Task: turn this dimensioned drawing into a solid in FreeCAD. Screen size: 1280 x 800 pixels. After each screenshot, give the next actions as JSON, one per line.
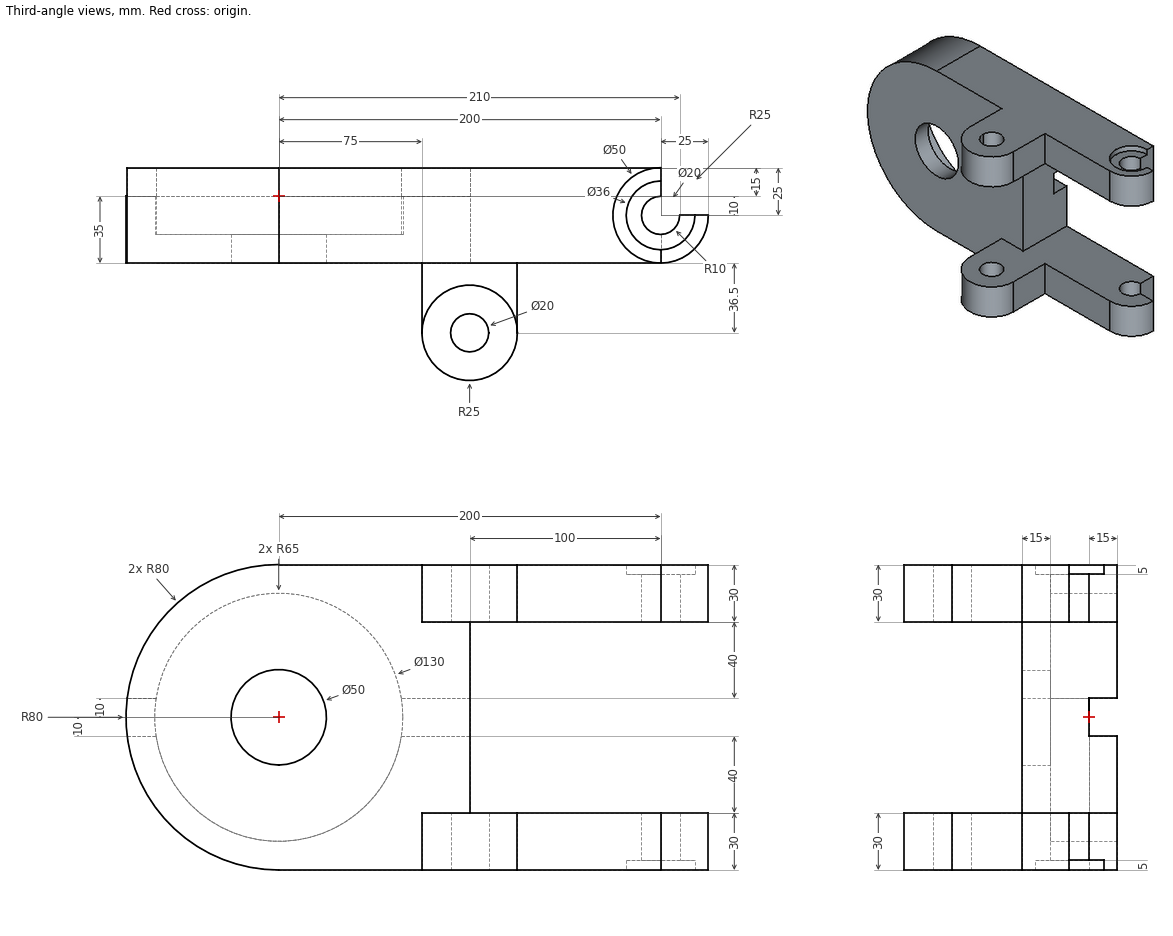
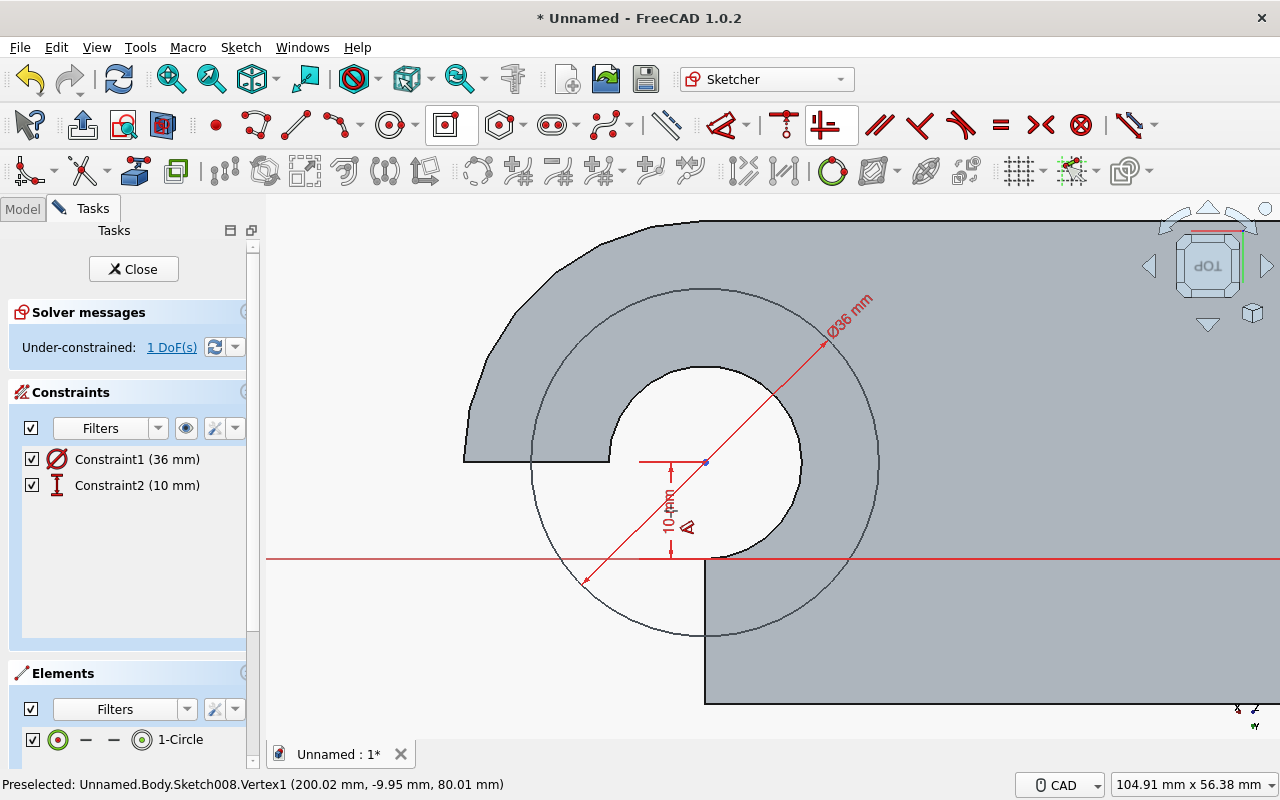
{"action": "left_click", "coordinate": [705, 462]}
{"action": "left_click", "coordinate": [910, 593]}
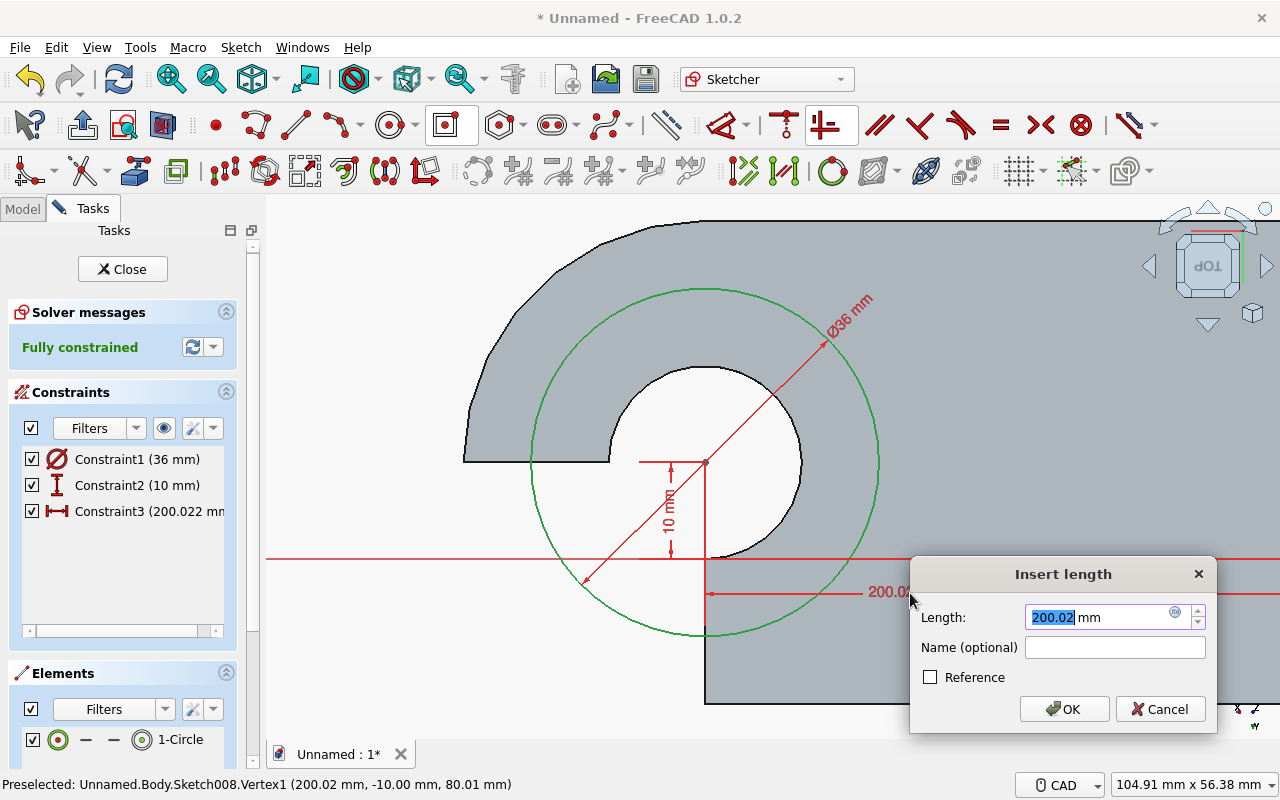
{"action": "type", "text": "200"}
{"action": "key", "text": "Return"}
{"action": "key", "text": "Escape"}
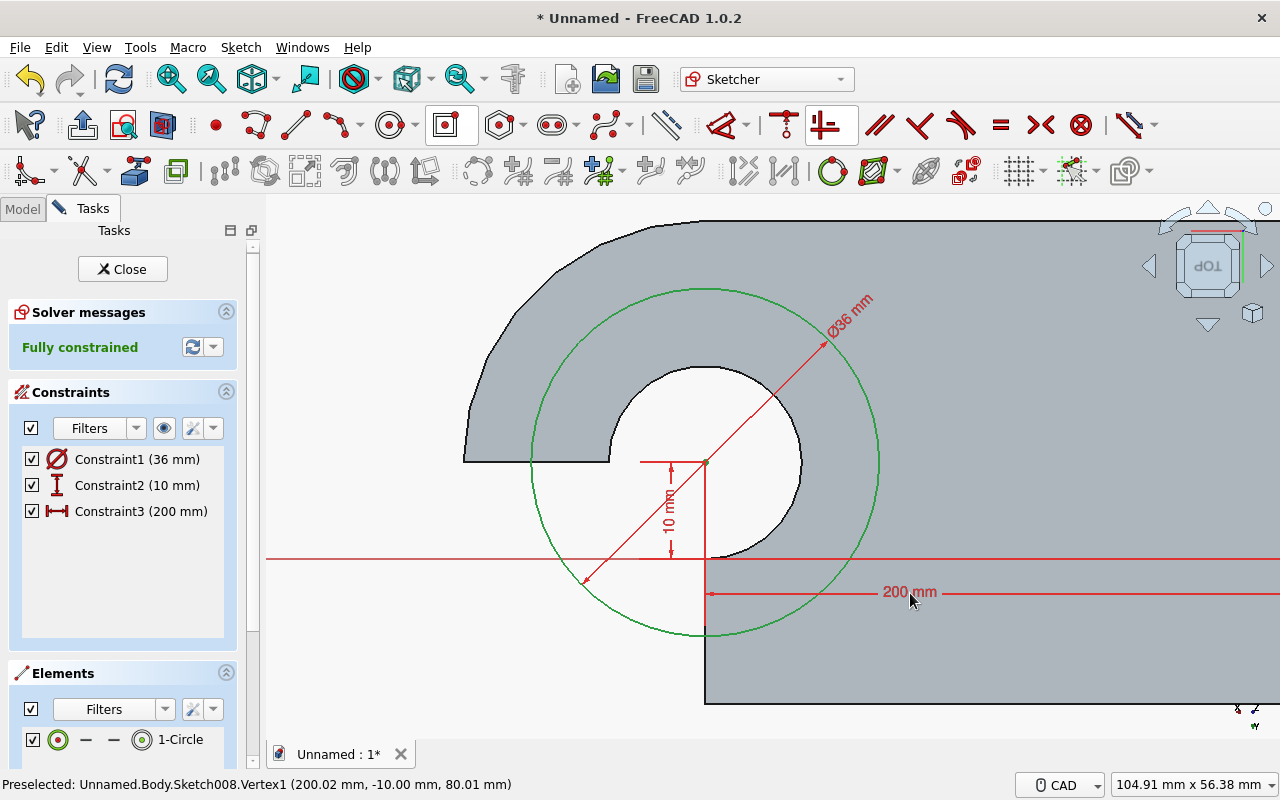
{"action": "left_click", "coordinate": [123, 269]}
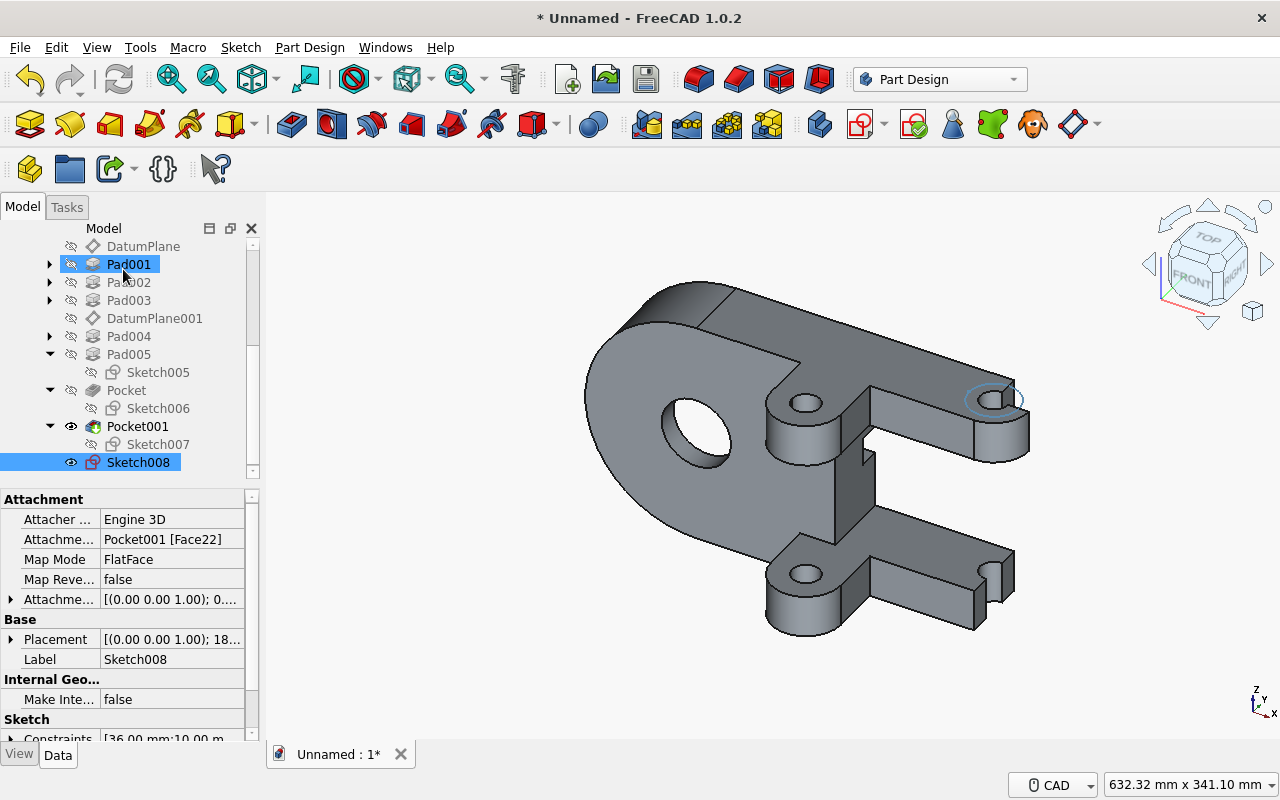
{"action": "left_click", "coordinate": [292, 124]}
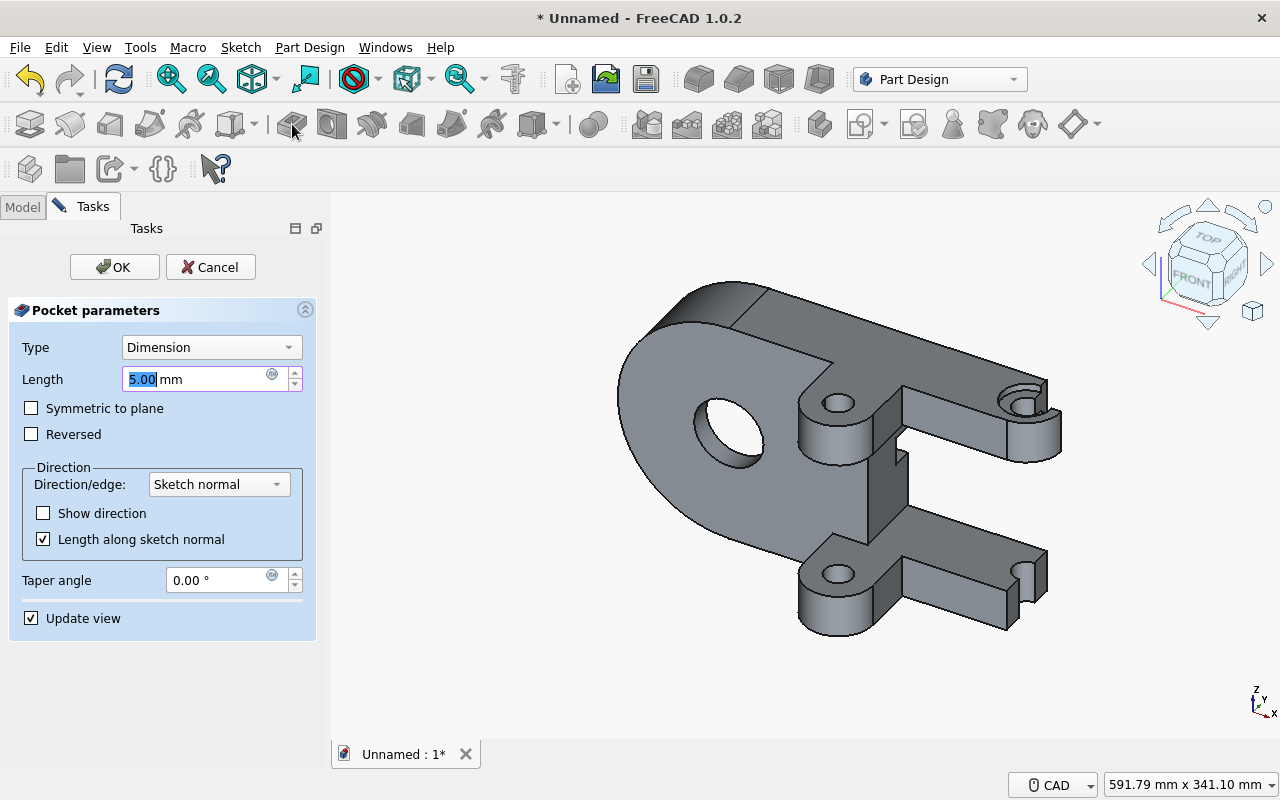
{"action": "type", "text": "5"}
{"action": "key", "text": "Tab"}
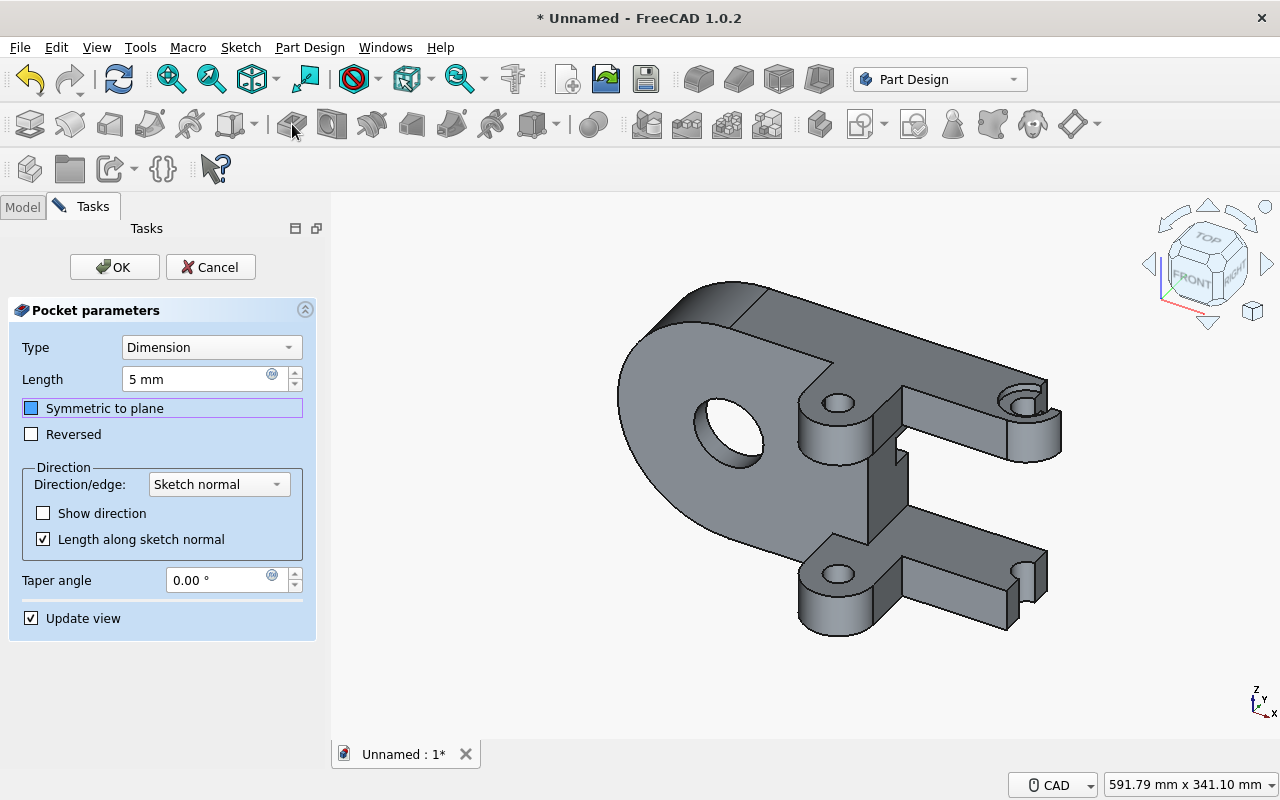
{"action": "left_click", "coordinate": [115, 267]}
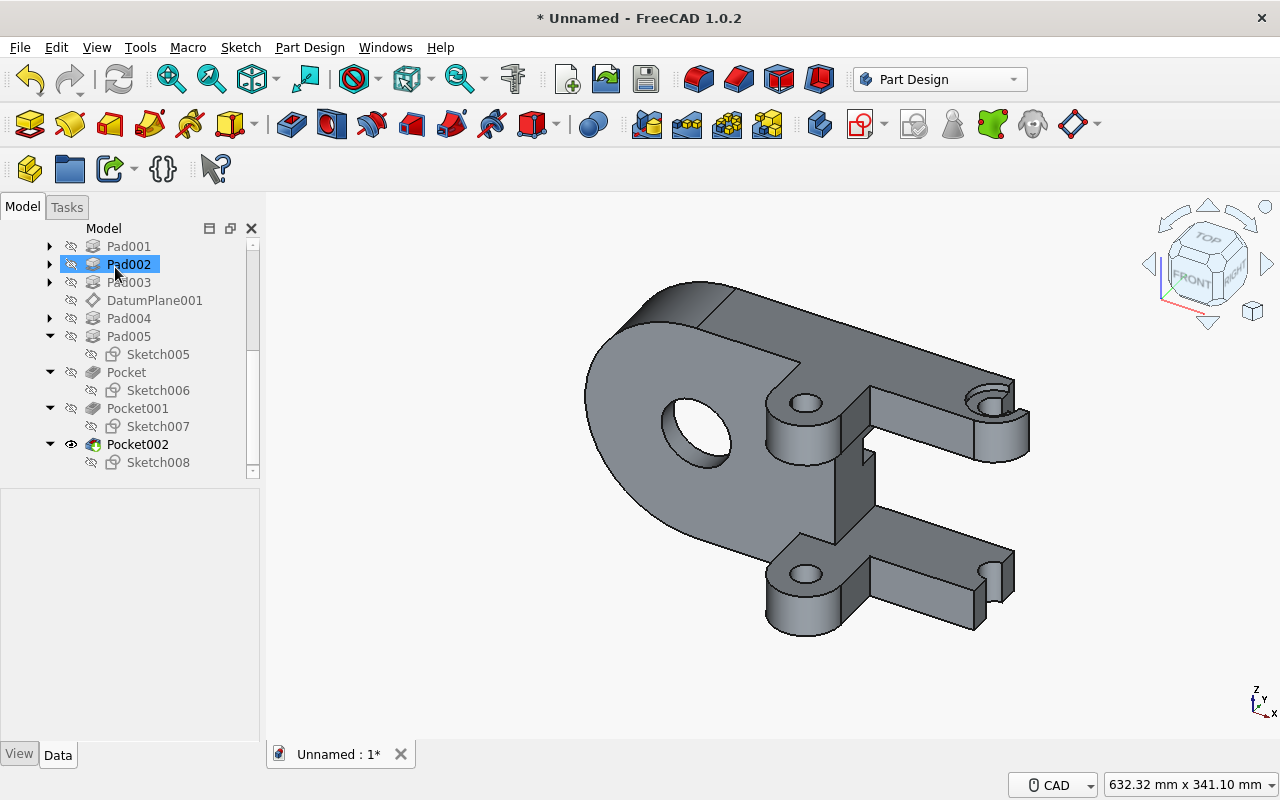
{"action": "scroll", "coordinate": [140, 350], "scroll_direction": "down", "scroll_amount": 3}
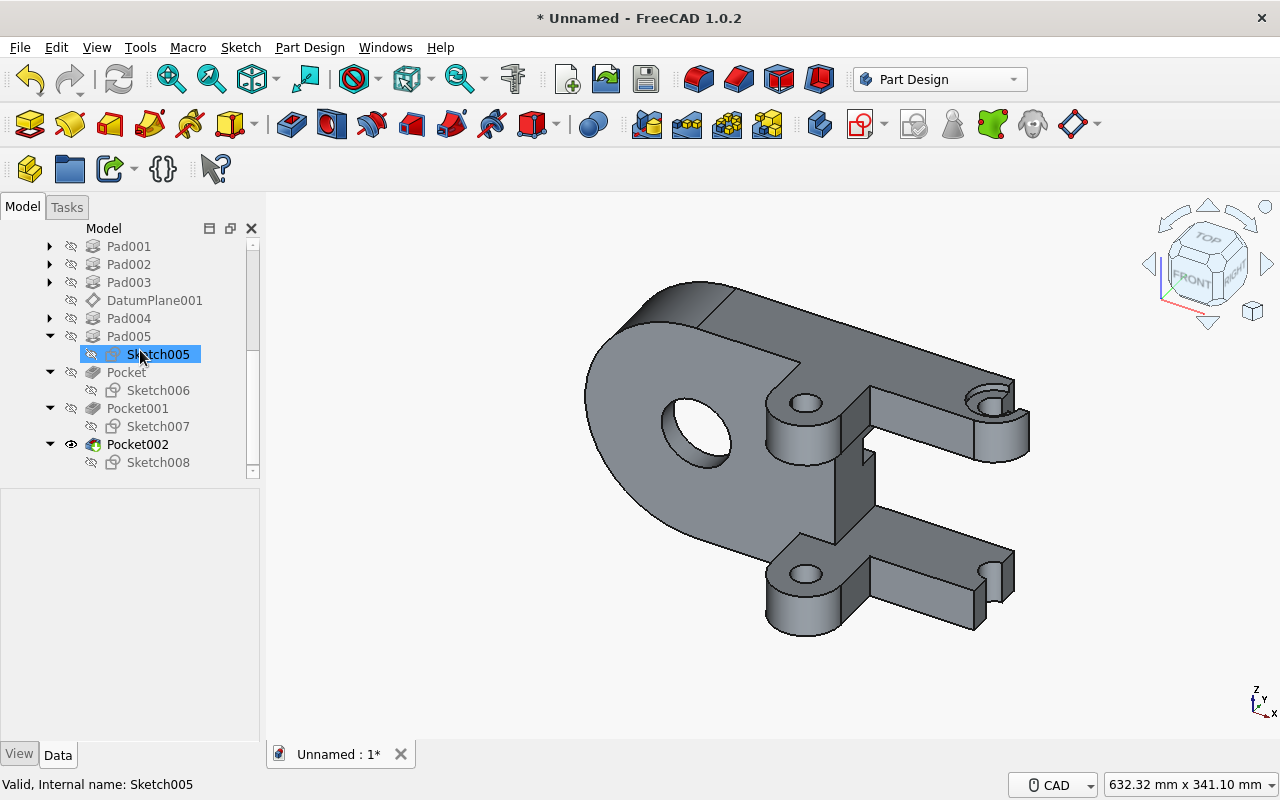
{"action": "scroll", "coordinate": [140, 350], "scroll_direction": "up", "scroll_amount": 15}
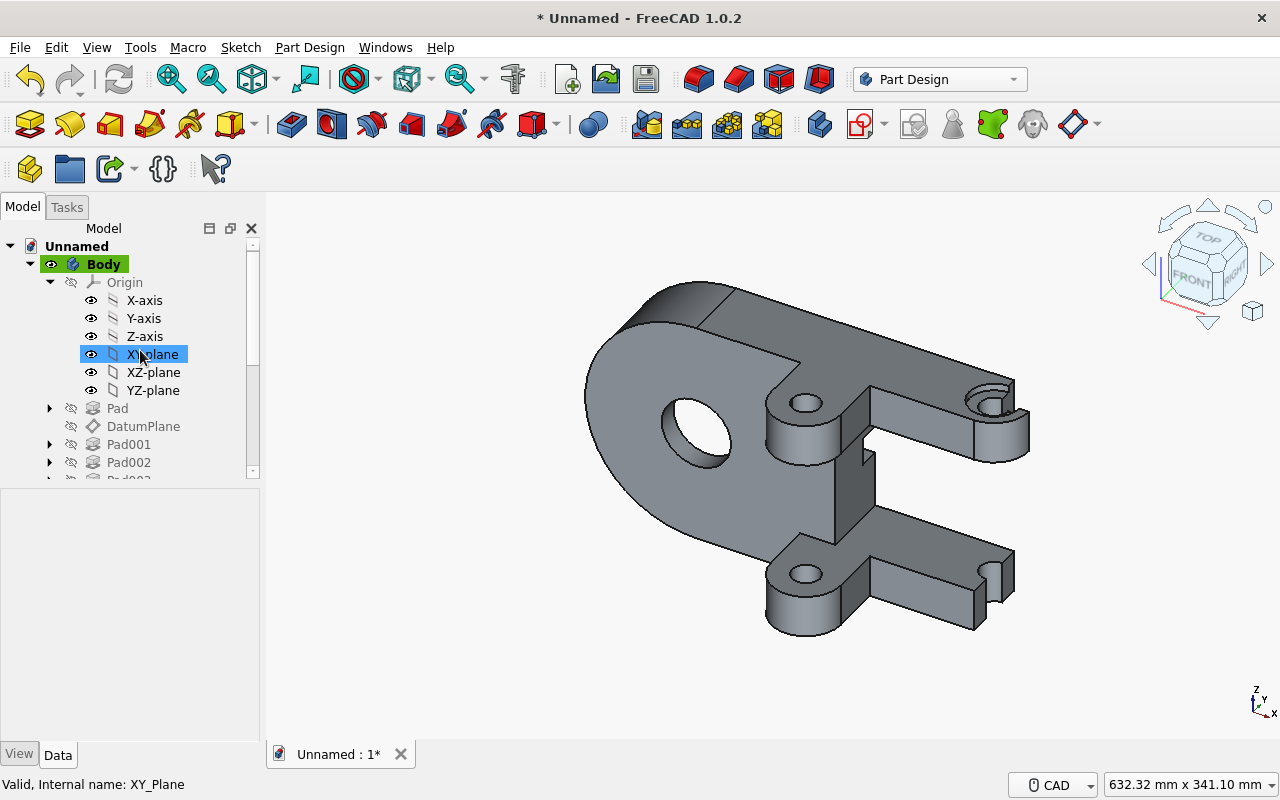
{"action": "left_click", "coordinate": [136, 354]}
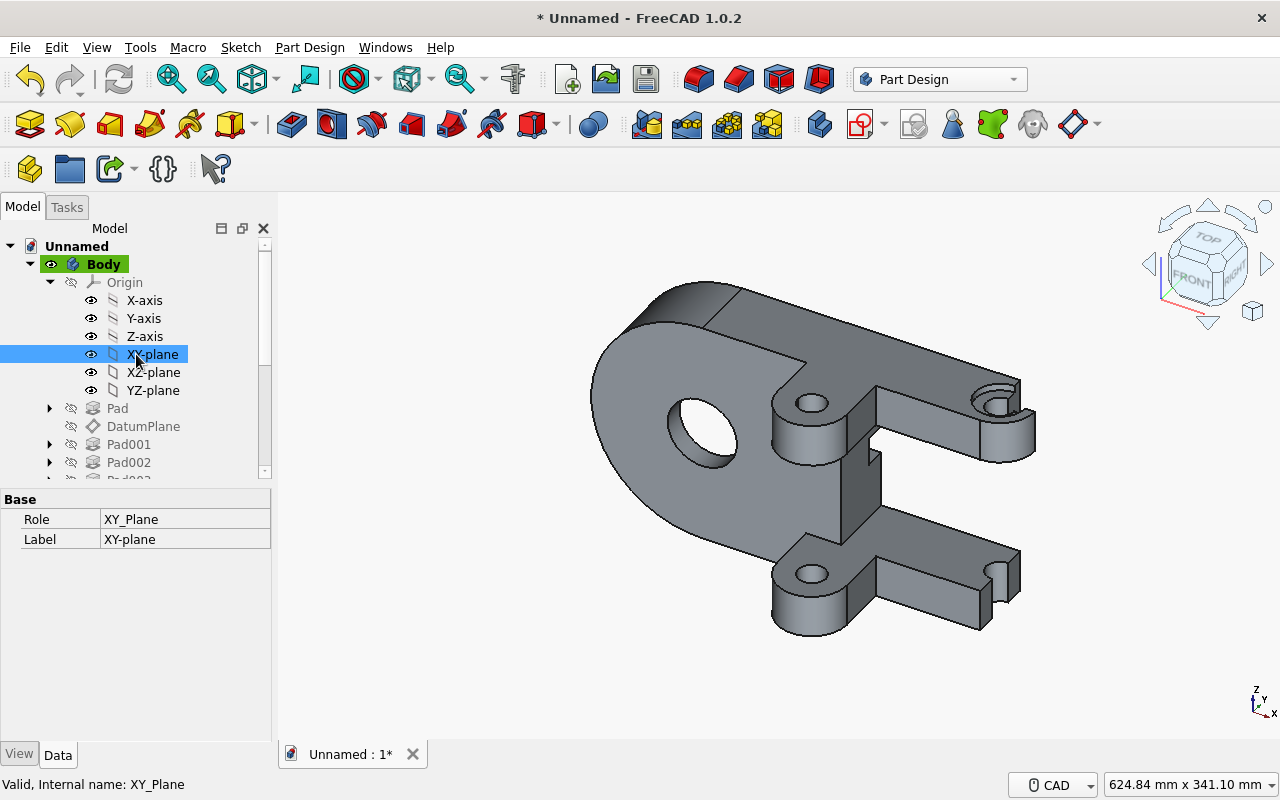
{"action": "left_click", "coordinate": [1074, 124]}